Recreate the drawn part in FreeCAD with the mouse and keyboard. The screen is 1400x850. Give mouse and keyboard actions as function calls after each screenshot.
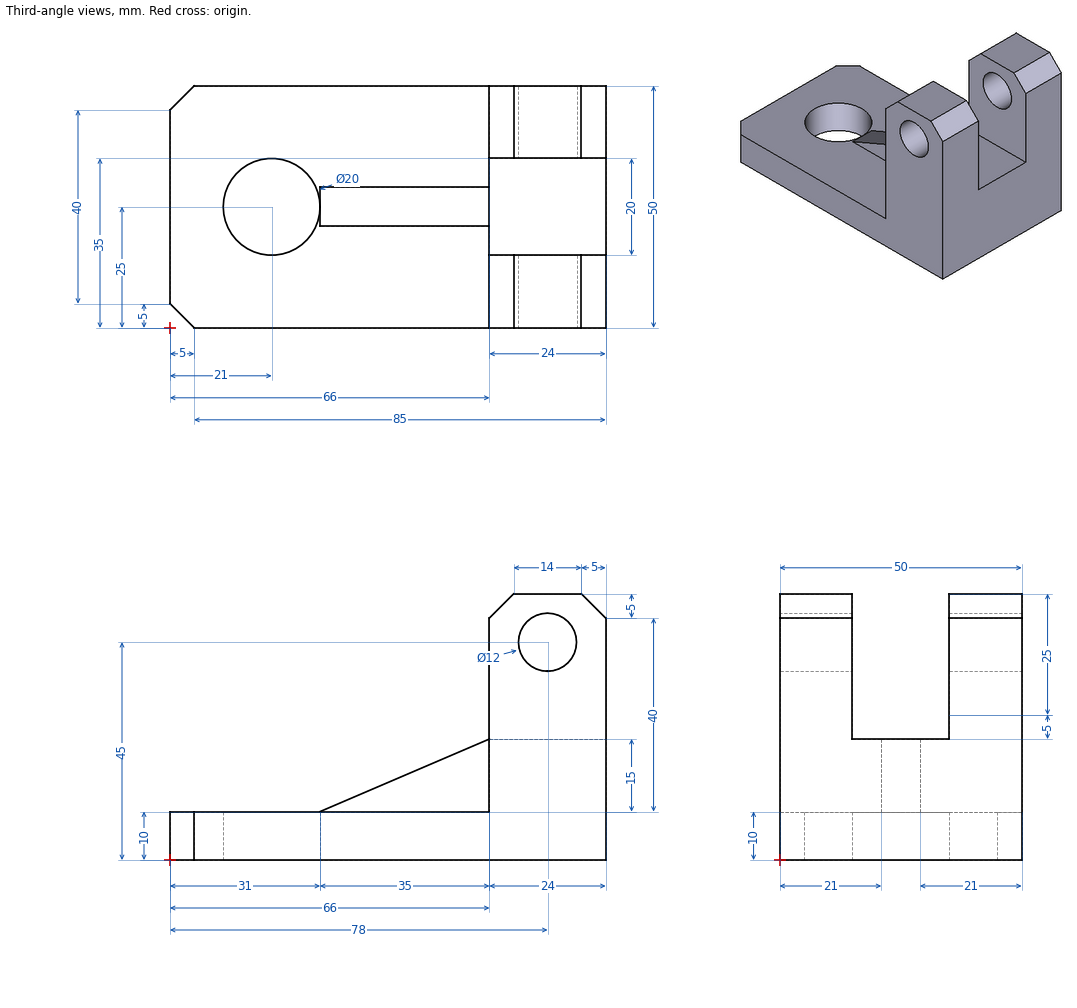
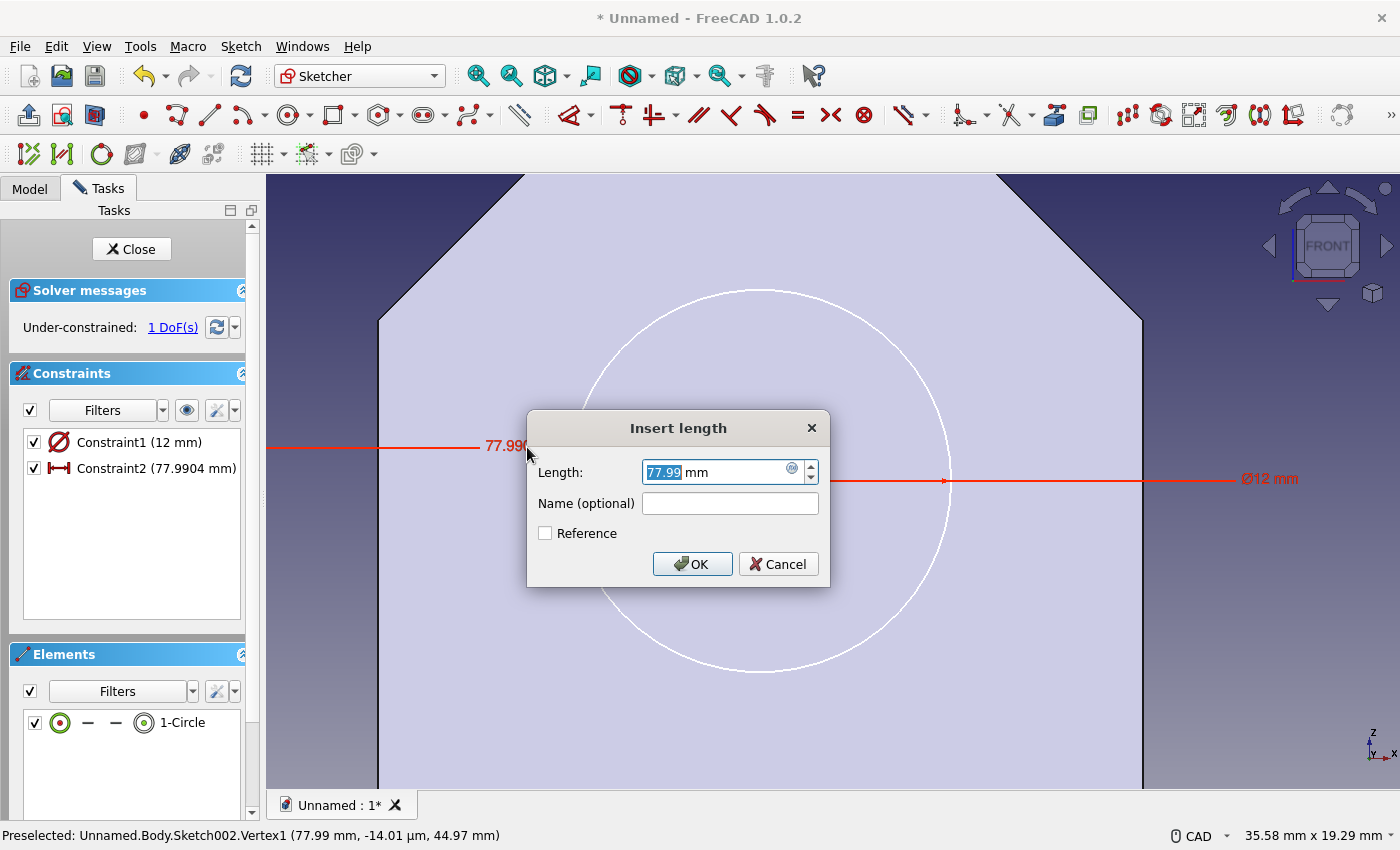
text(78)
key(Return)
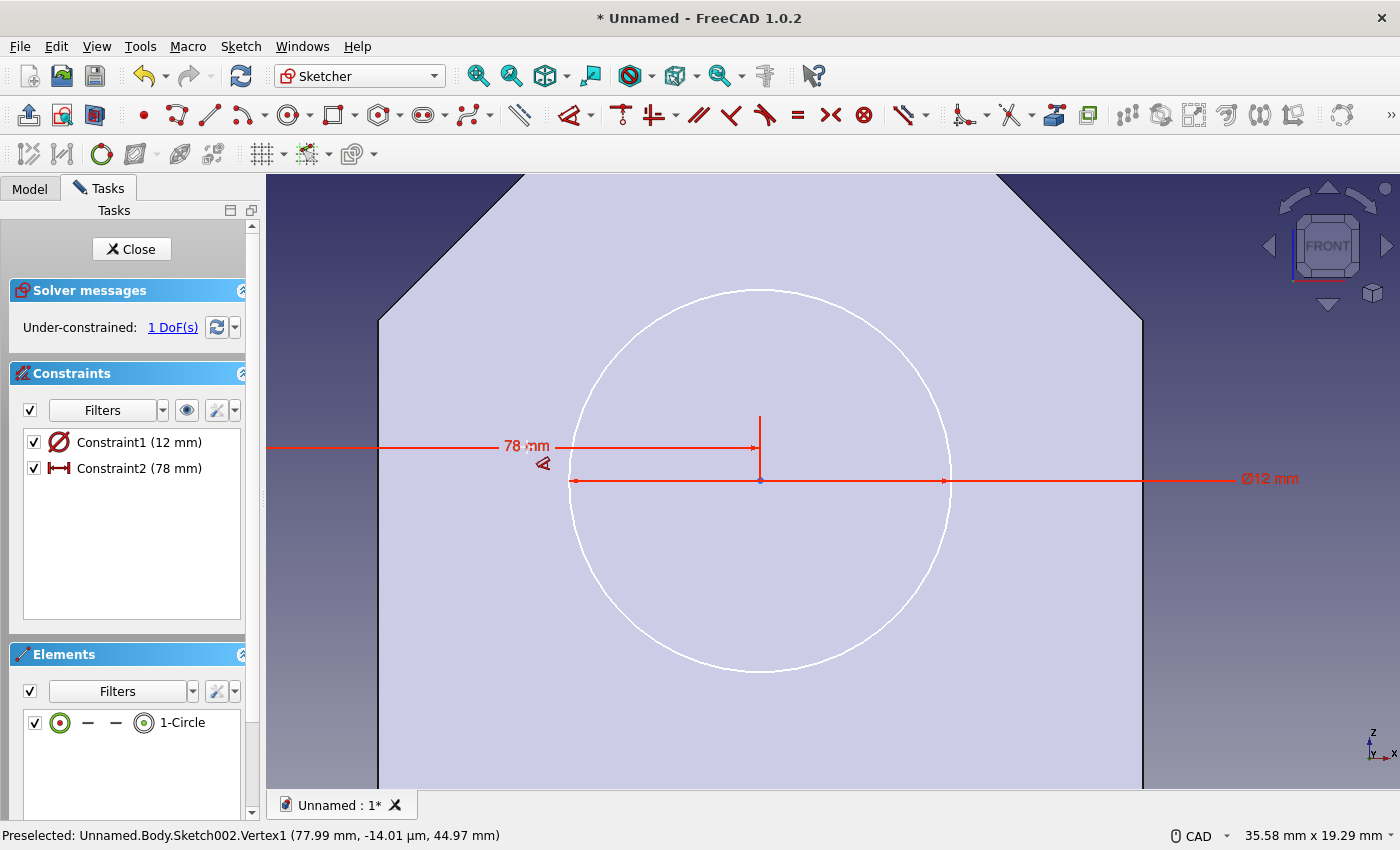
click(760, 481)
click(794, 621)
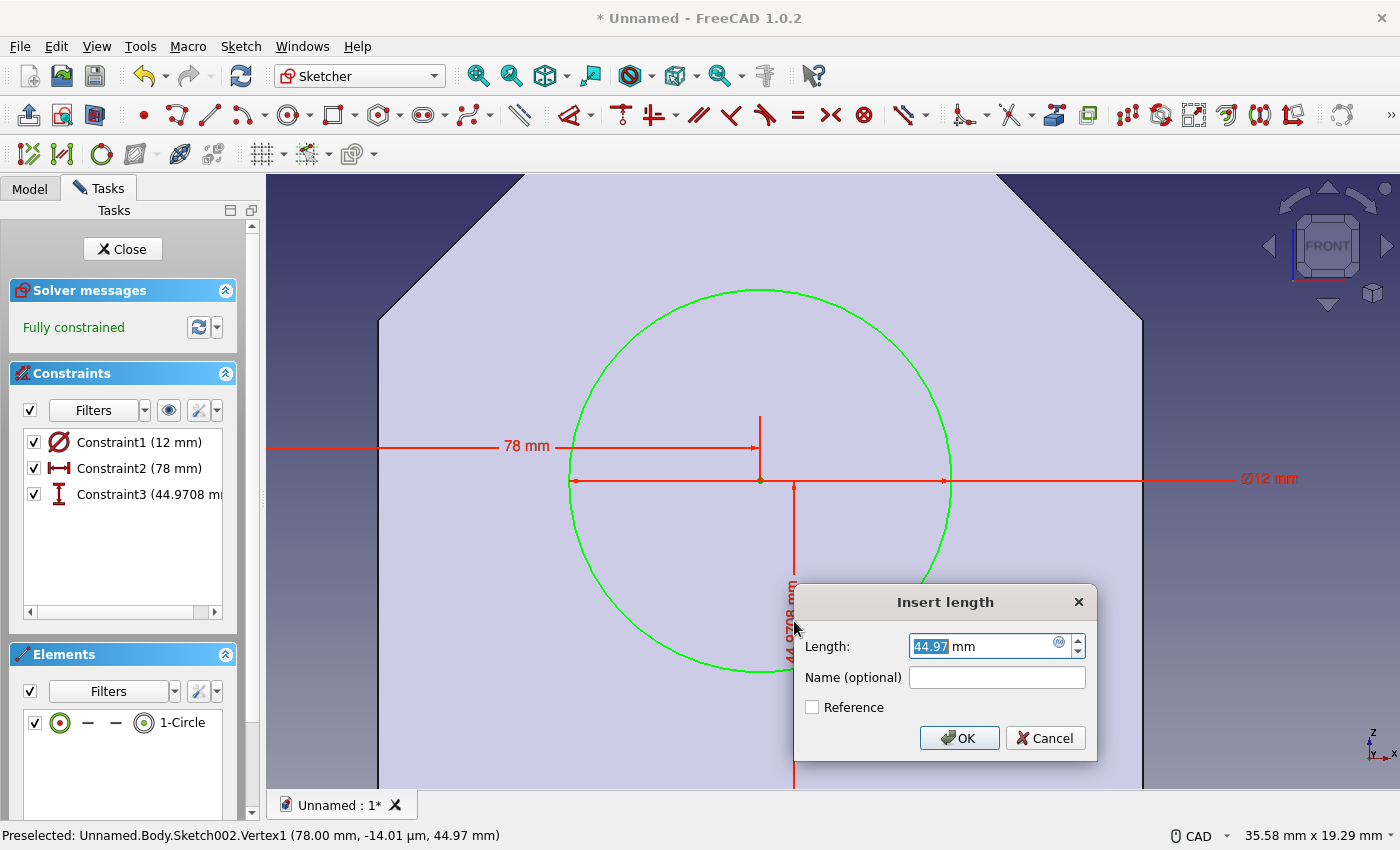
text(45)
key(Return)
key(Escape)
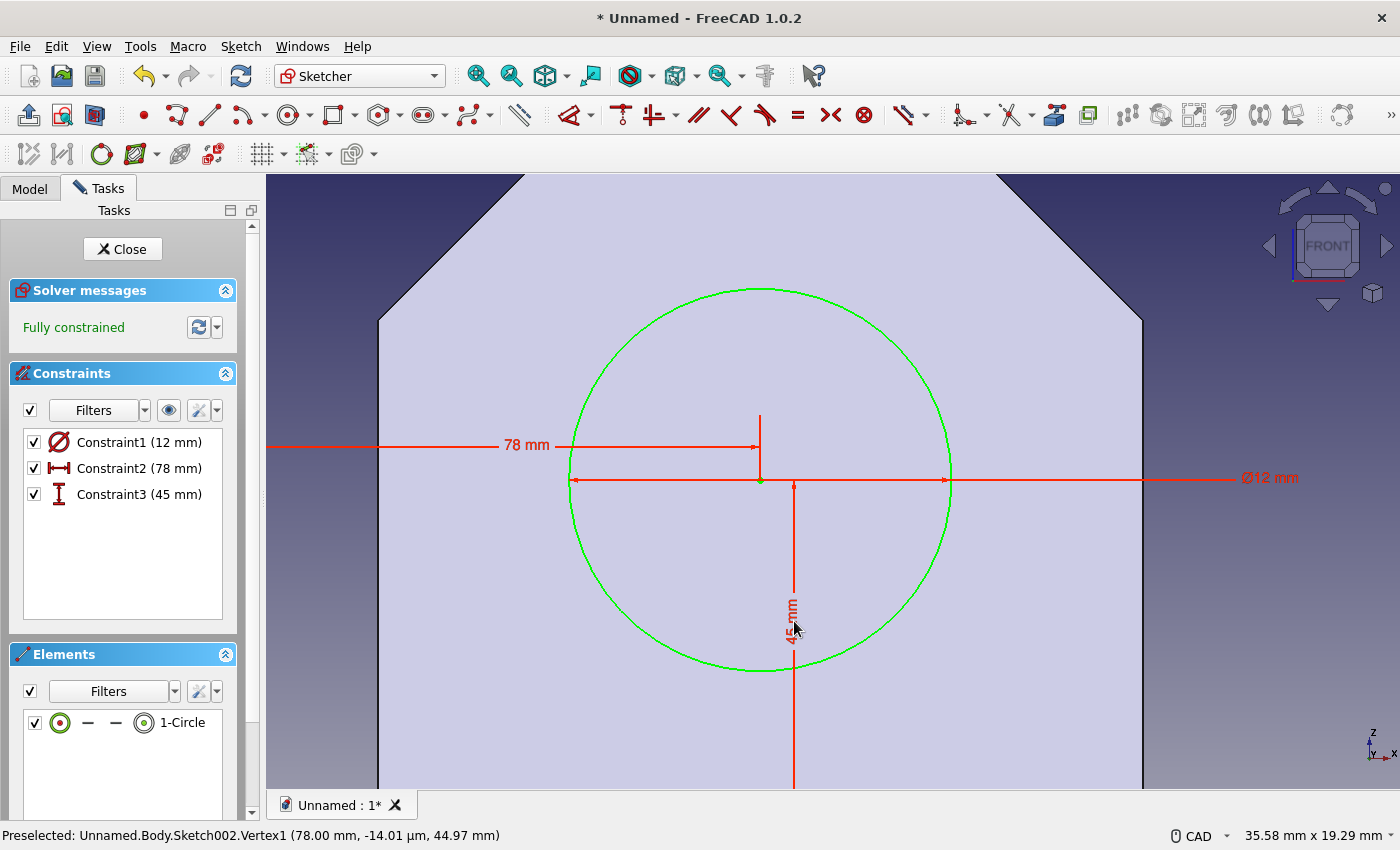
click(123, 249)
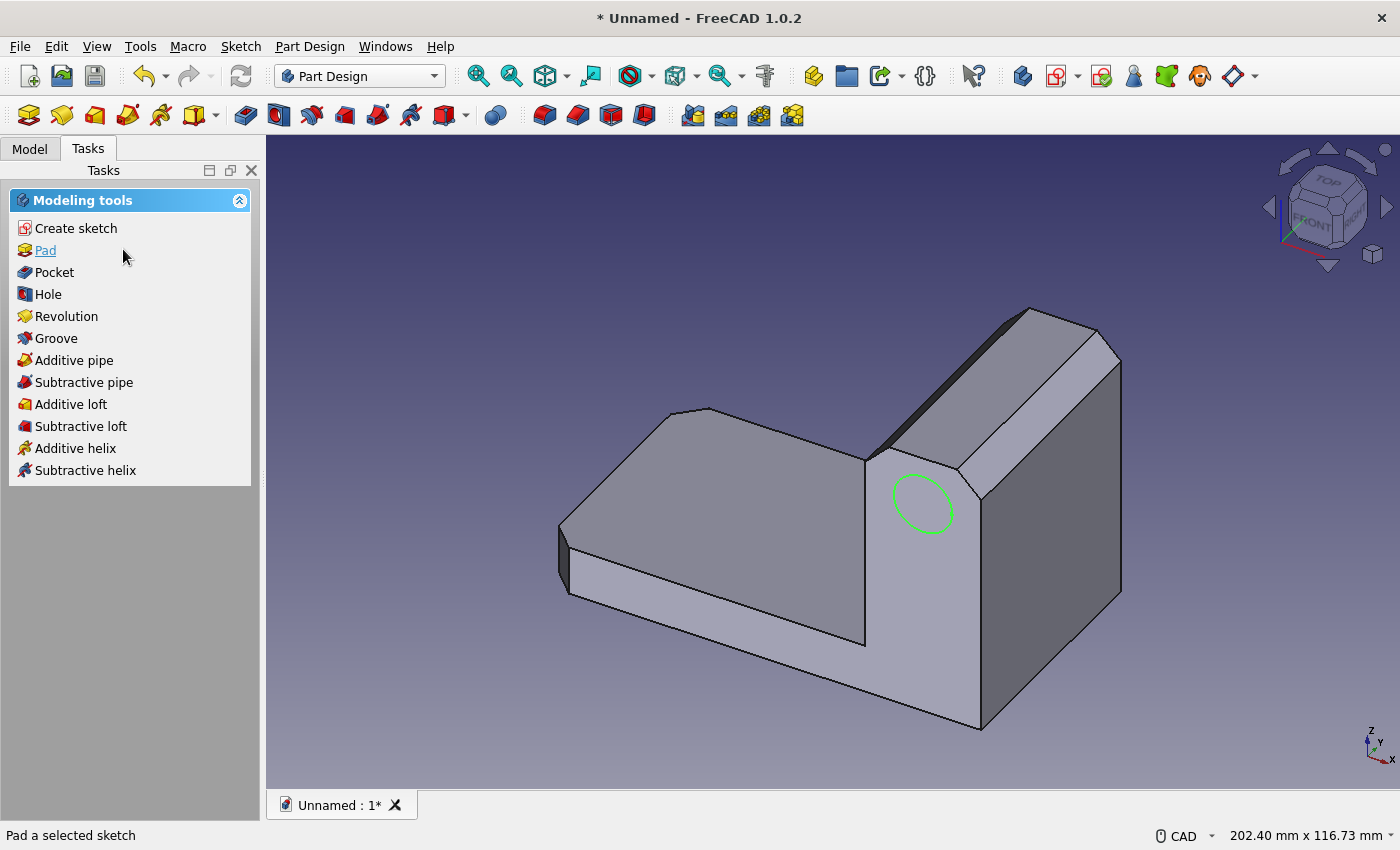
click(246, 116)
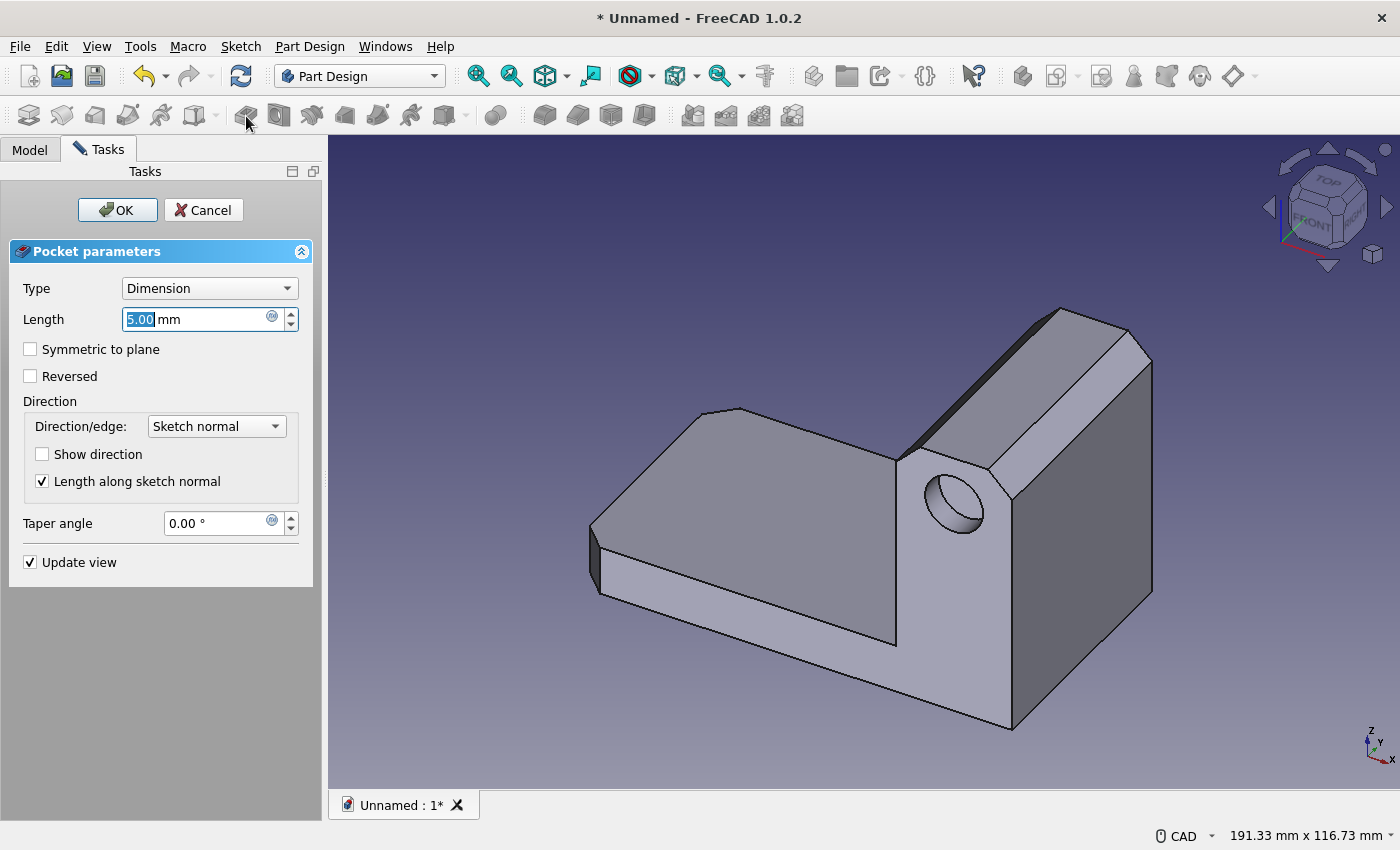
text(50)
key(Tab)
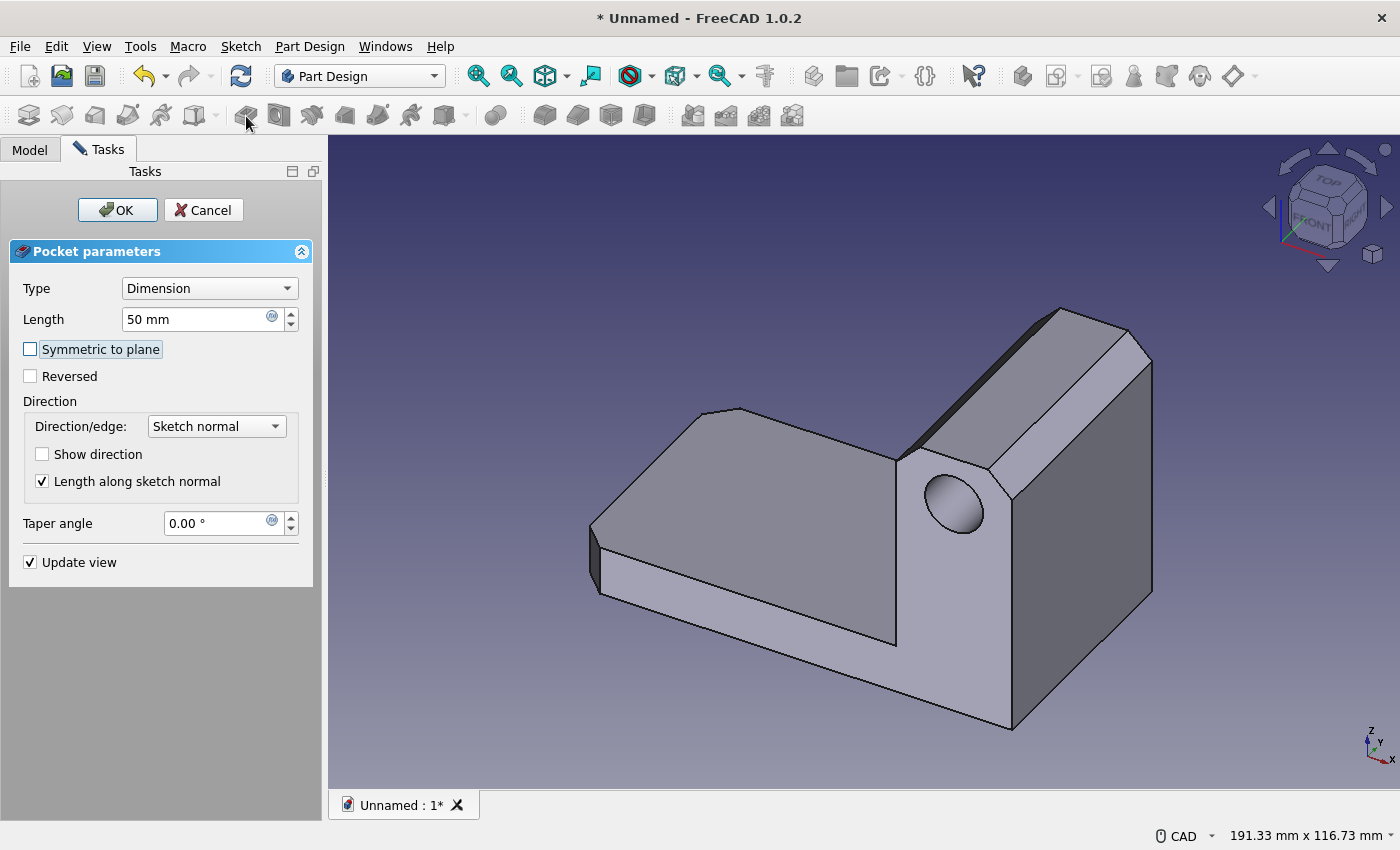
click(118, 210)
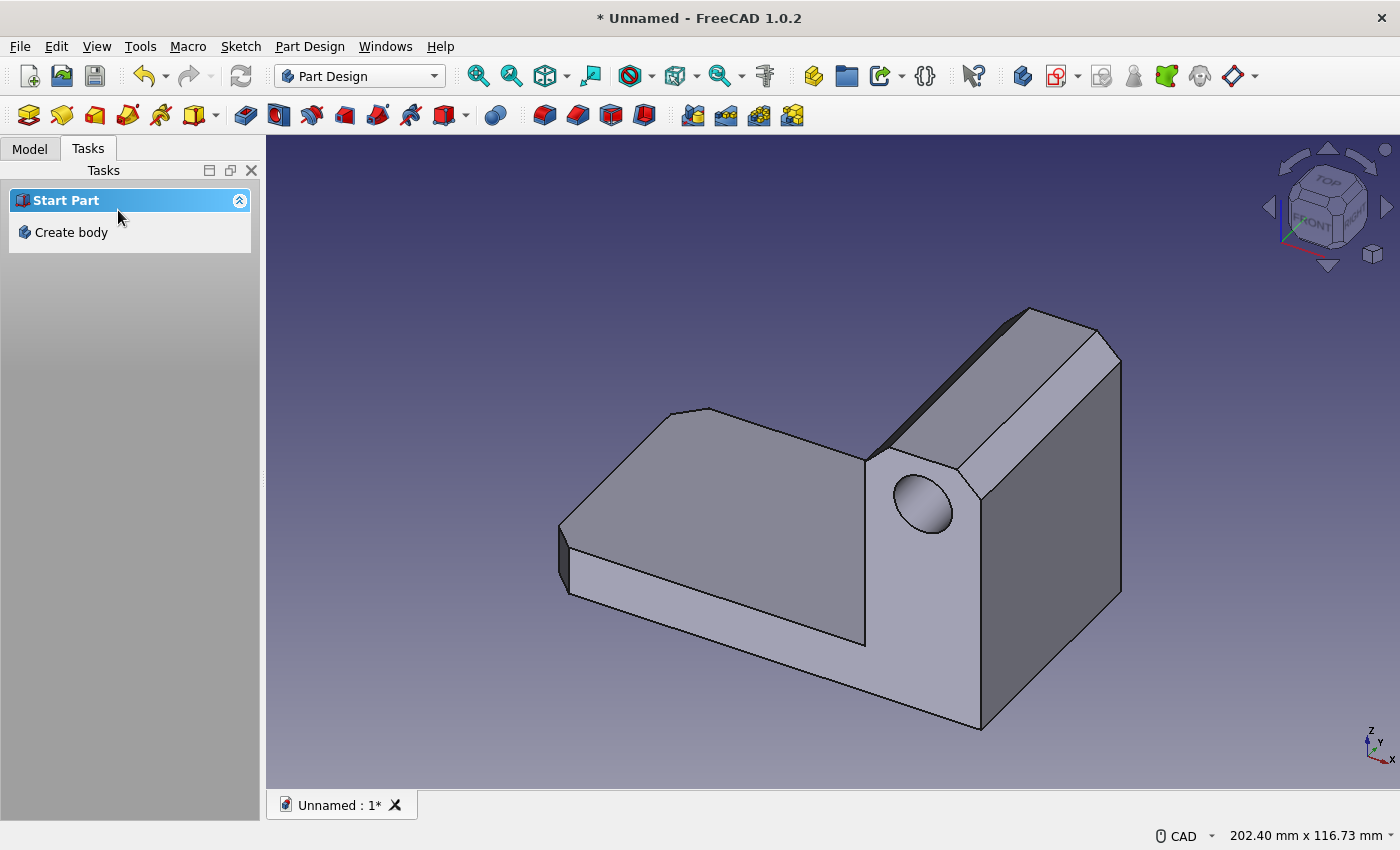
click(1033, 348)